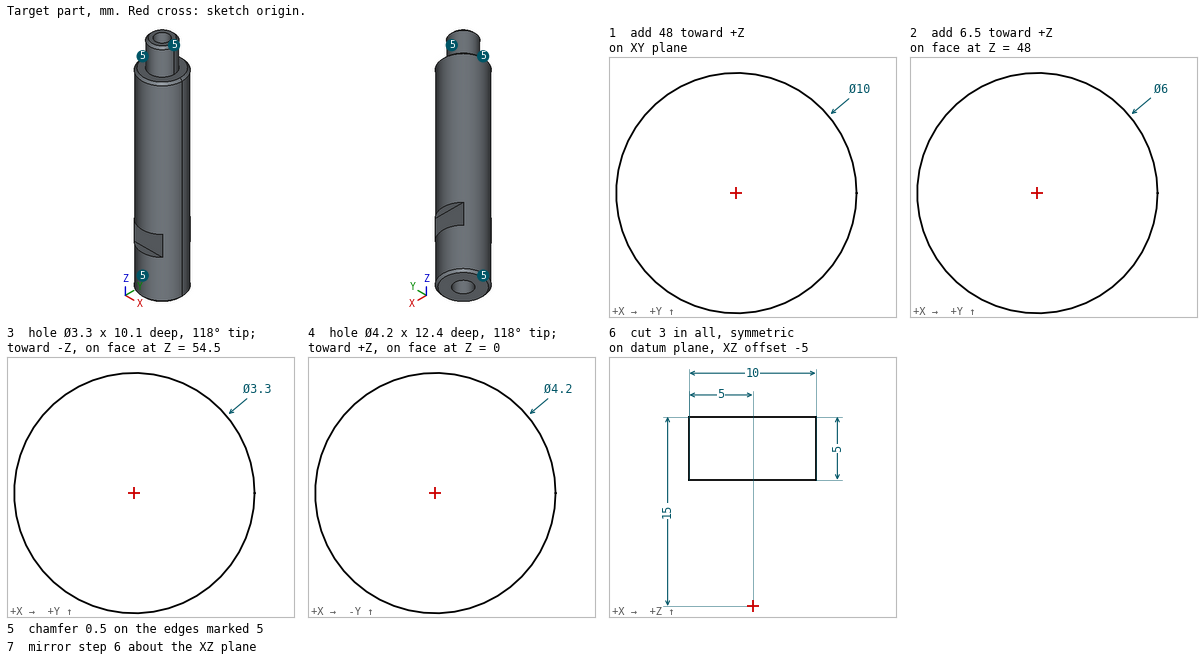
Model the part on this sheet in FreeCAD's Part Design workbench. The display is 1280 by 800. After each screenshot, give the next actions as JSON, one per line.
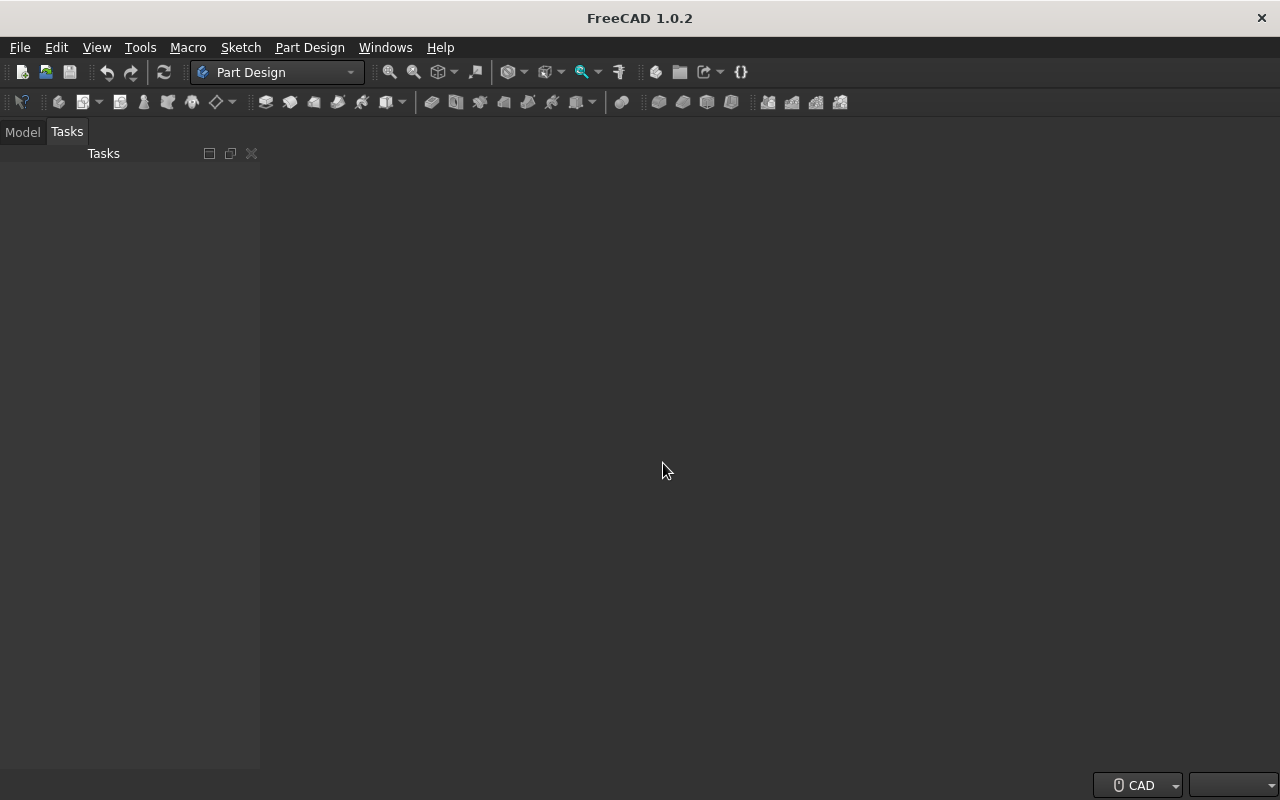
{"action": "left_click", "coordinate": [22, 72]}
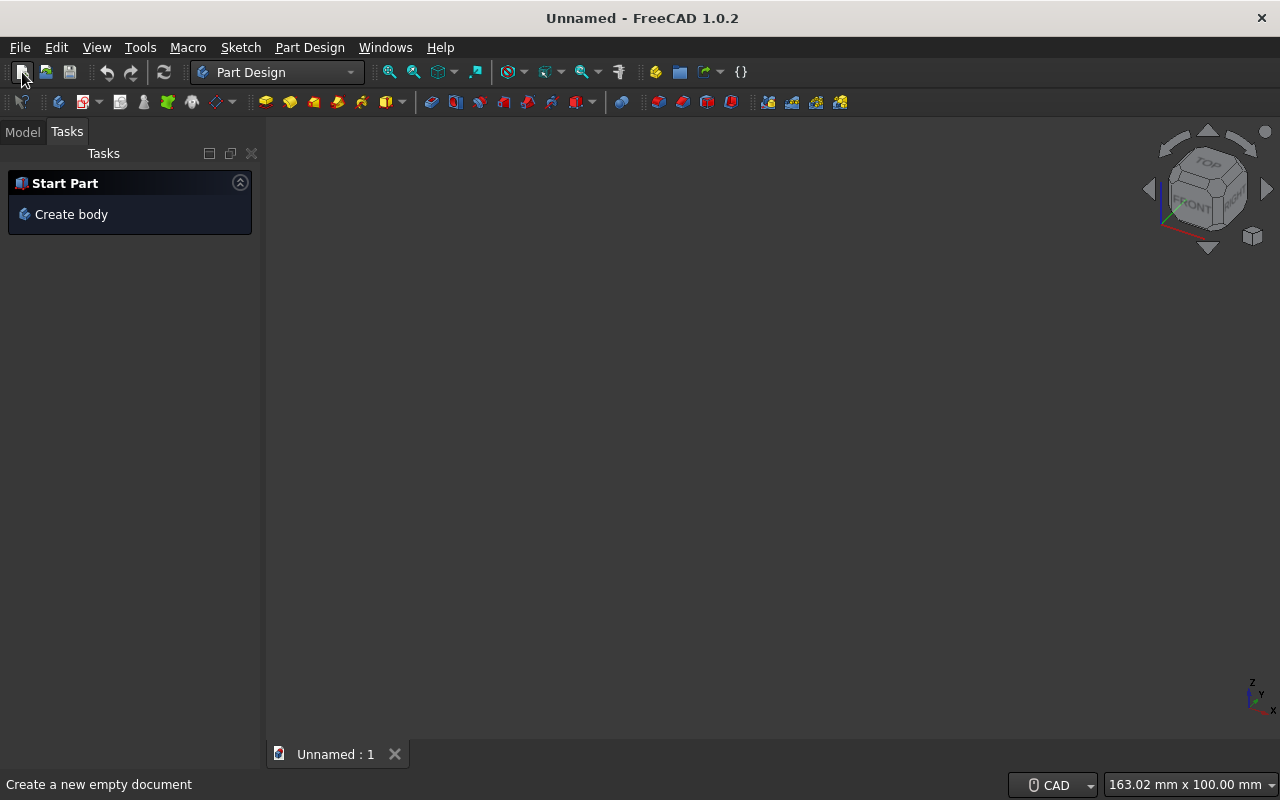
{"action": "left_click", "coordinate": [84, 102]}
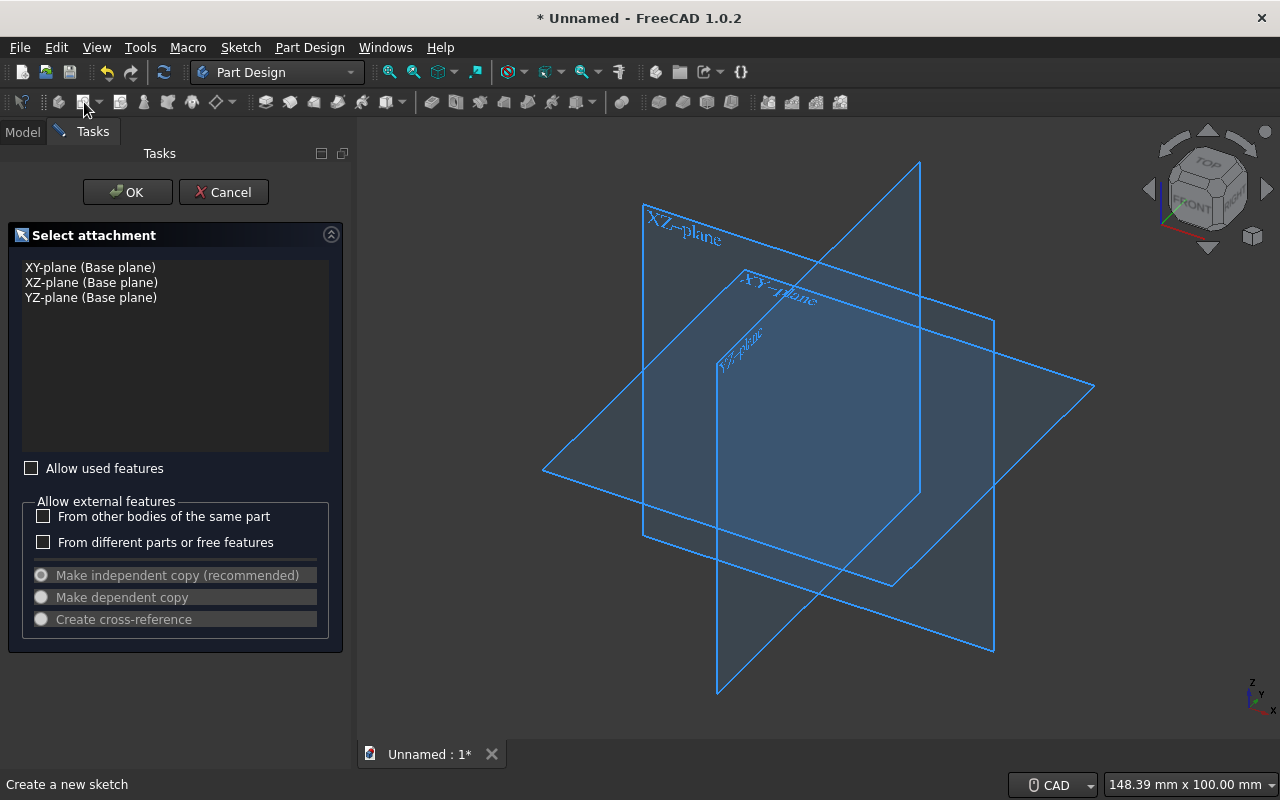
{"action": "left_click", "coordinate": [82, 268]}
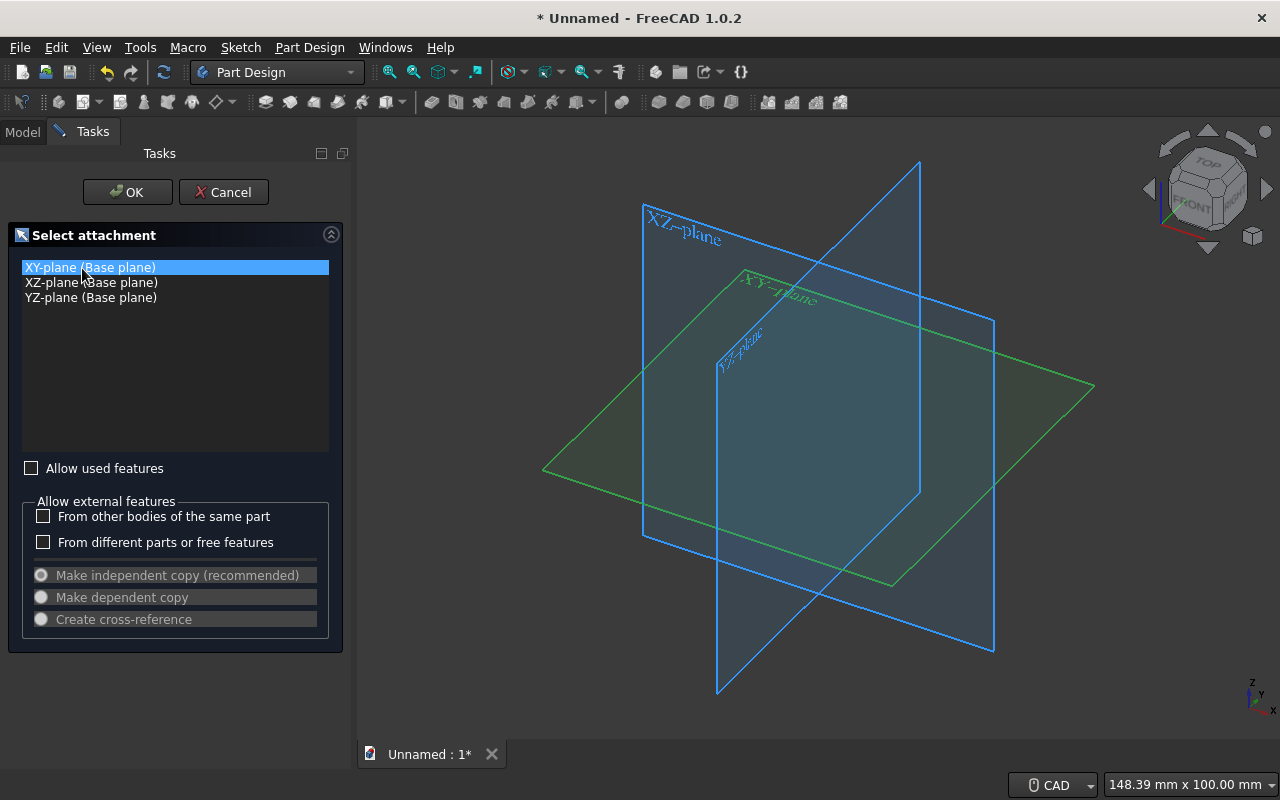
{"action": "left_click", "coordinate": [128, 192]}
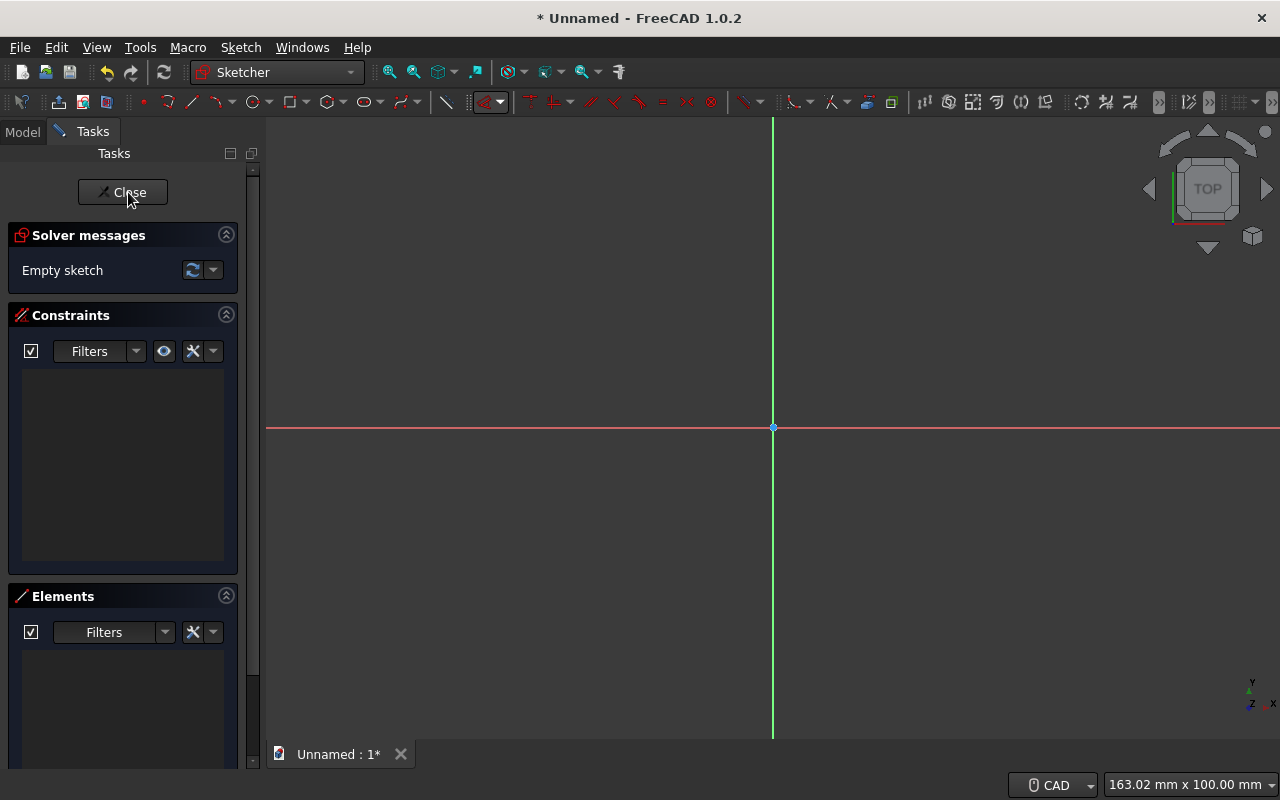
{"action": "scroll", "coordinate": [787, 428], "scroll_direction": "up", "scroll_amount": 9}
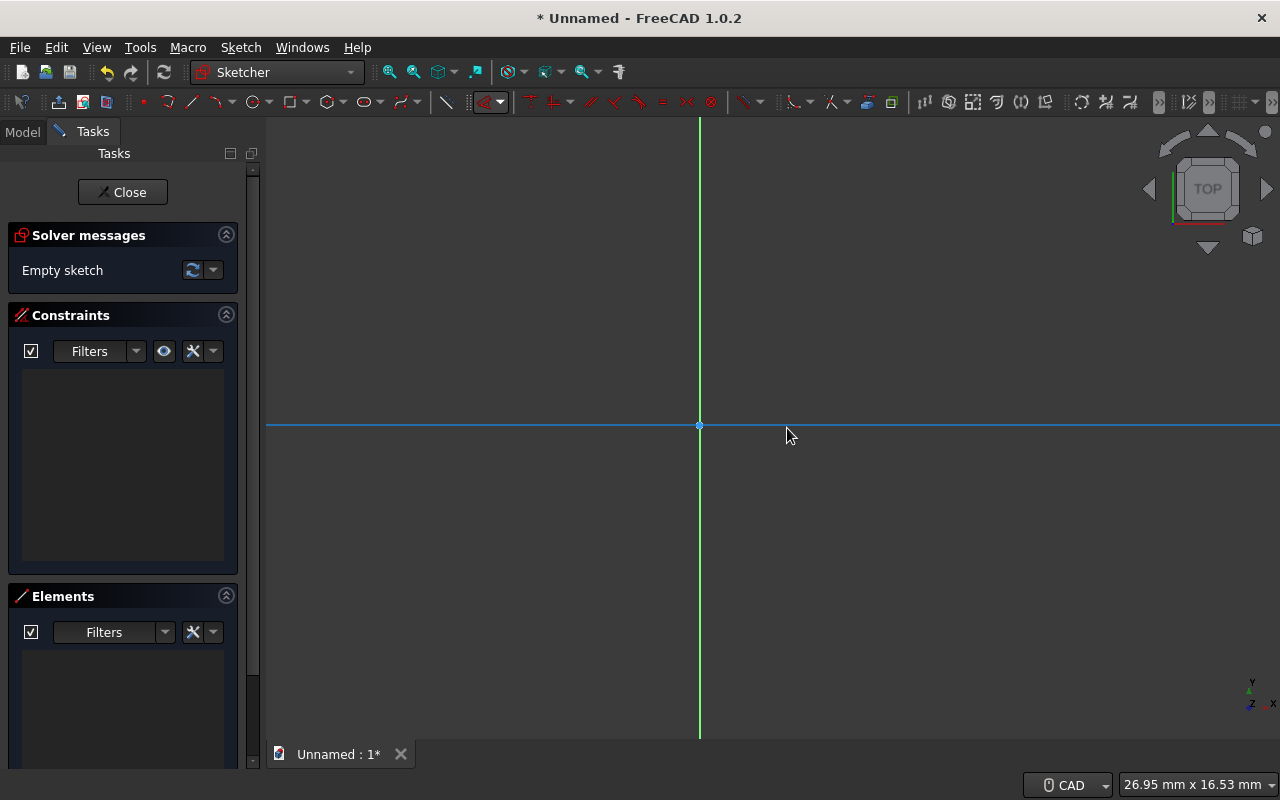
{"action": "left_click", "coordinate": [254, 102]}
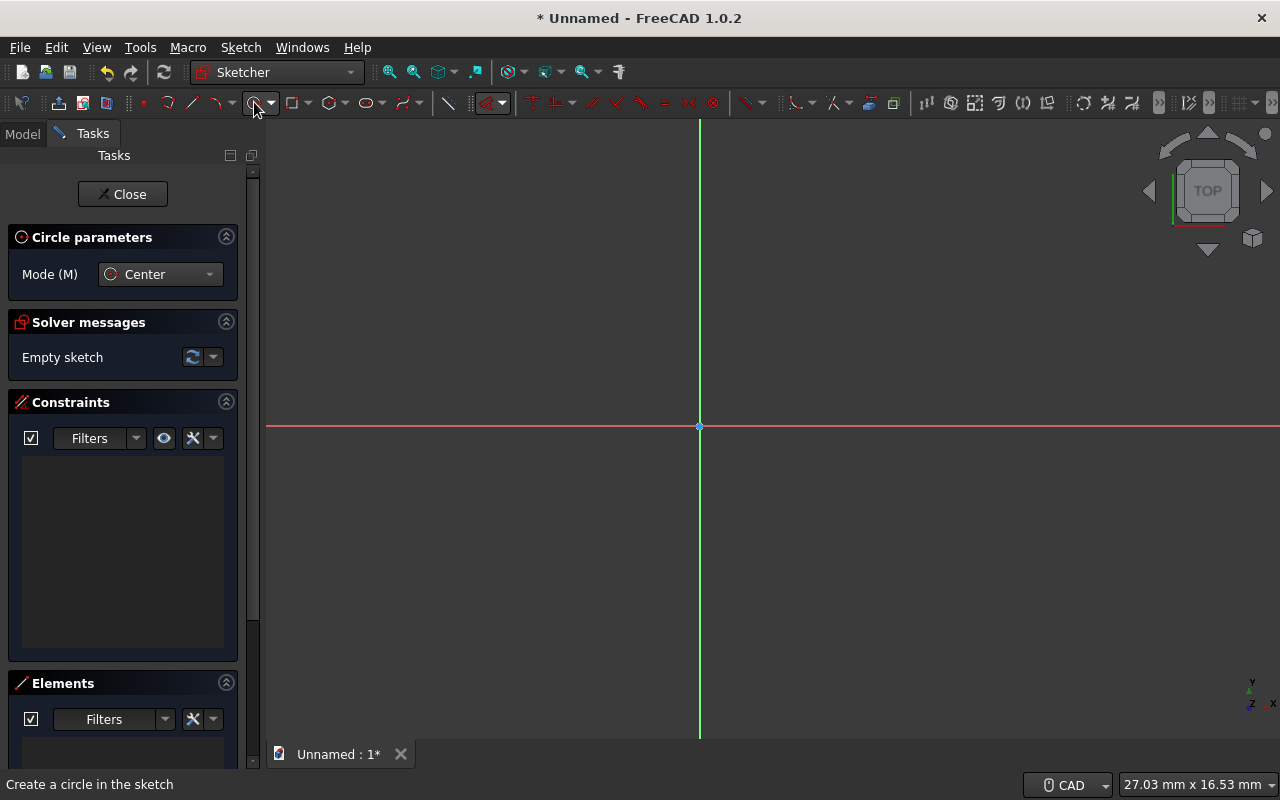
{"action": "left_click", "coordinate": [700, 426]}
{"action": "mouse_move", "coordinate": [833, 294]}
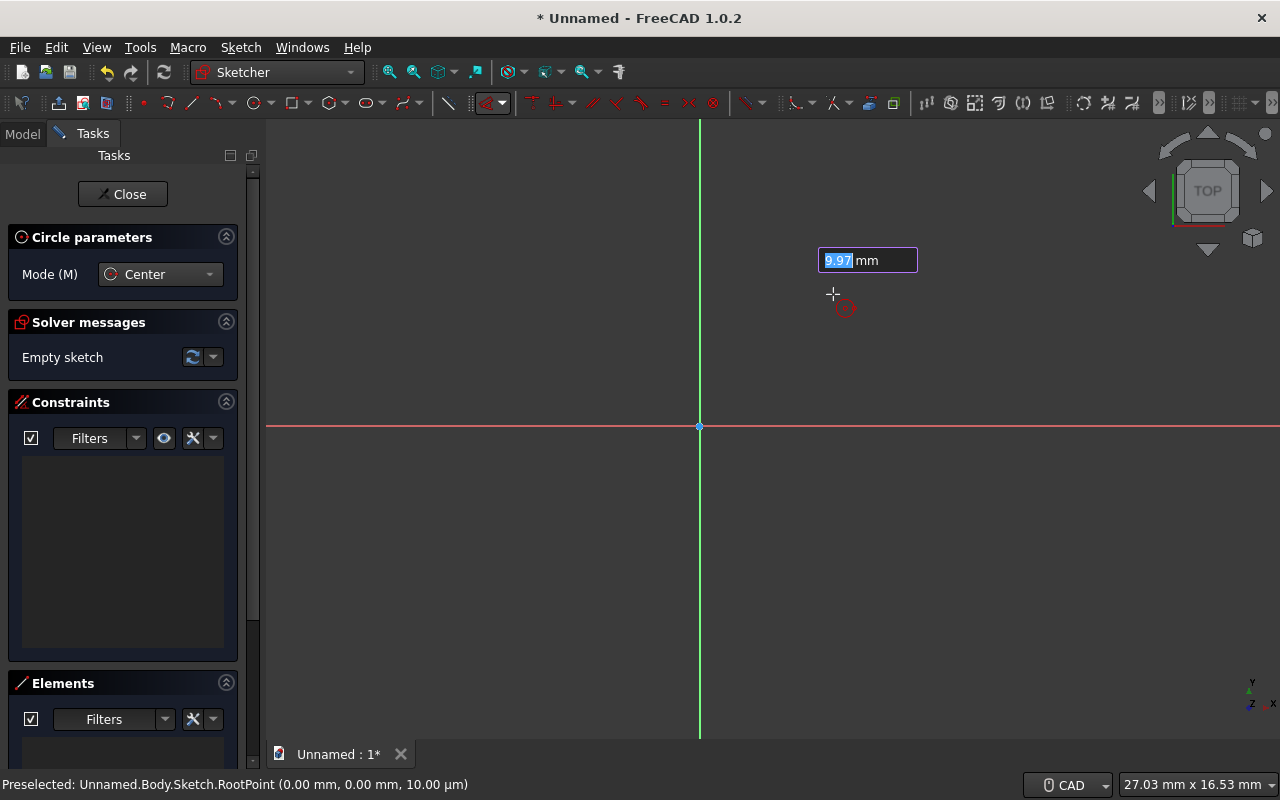
{"action": "type", "text": "10"}
{"action": "key", "text": "Return"}
{"action": "key", "text": "Escape"}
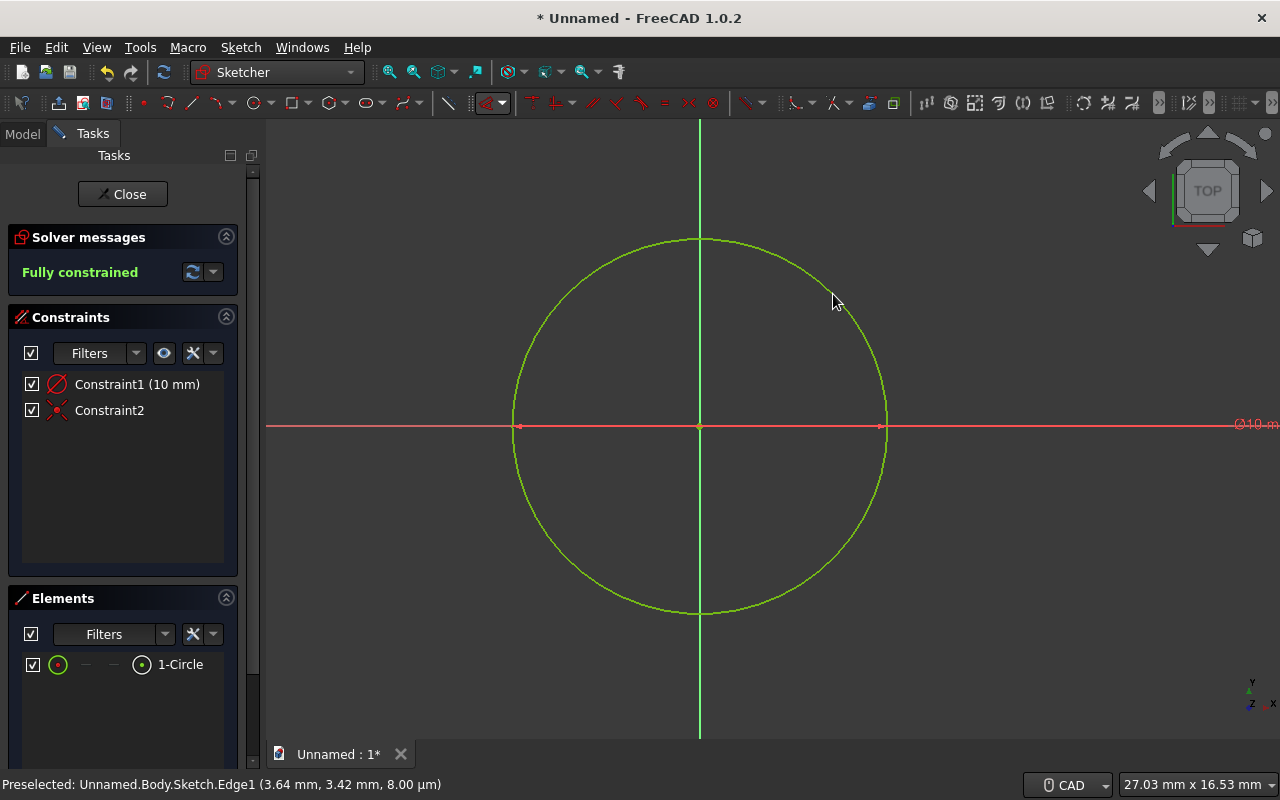
{"action": "left_click", "coordinate": [123, 194]}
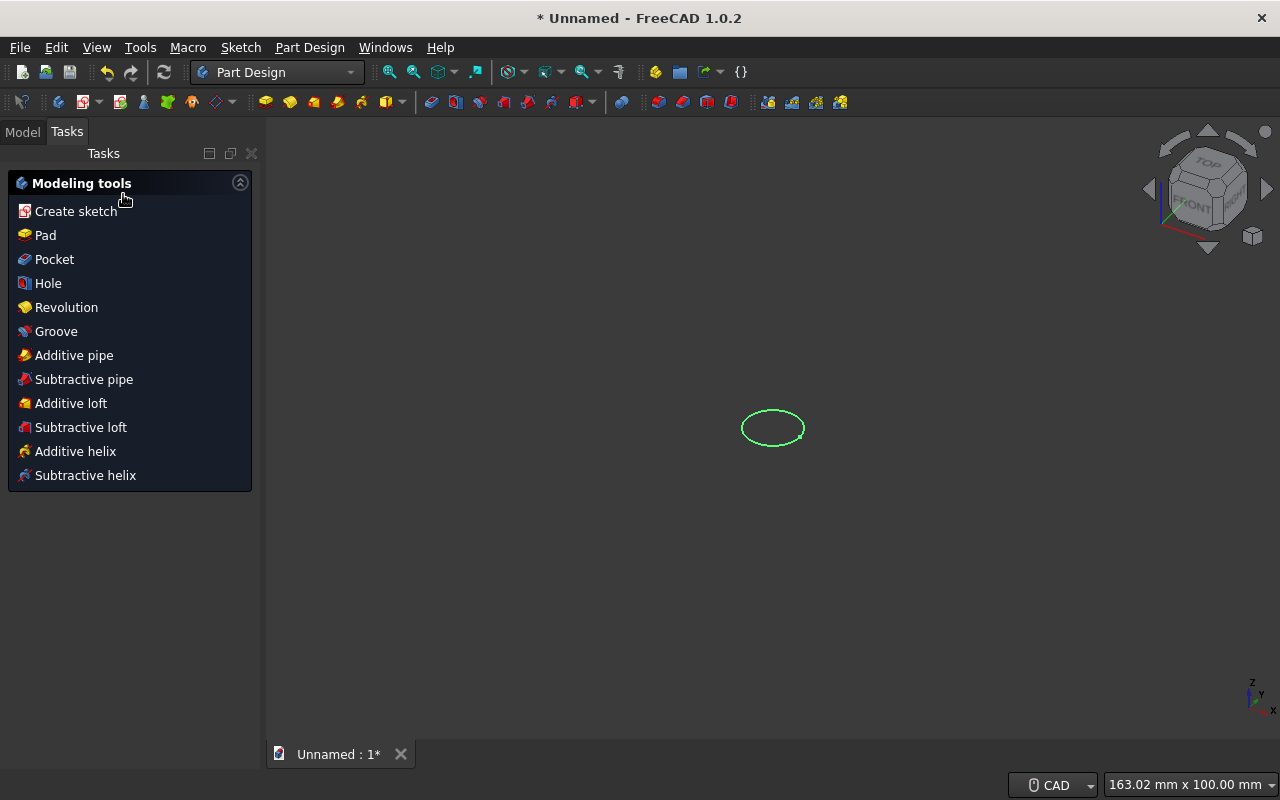
{"action": "left_click", "coordinate": [266, 102]}